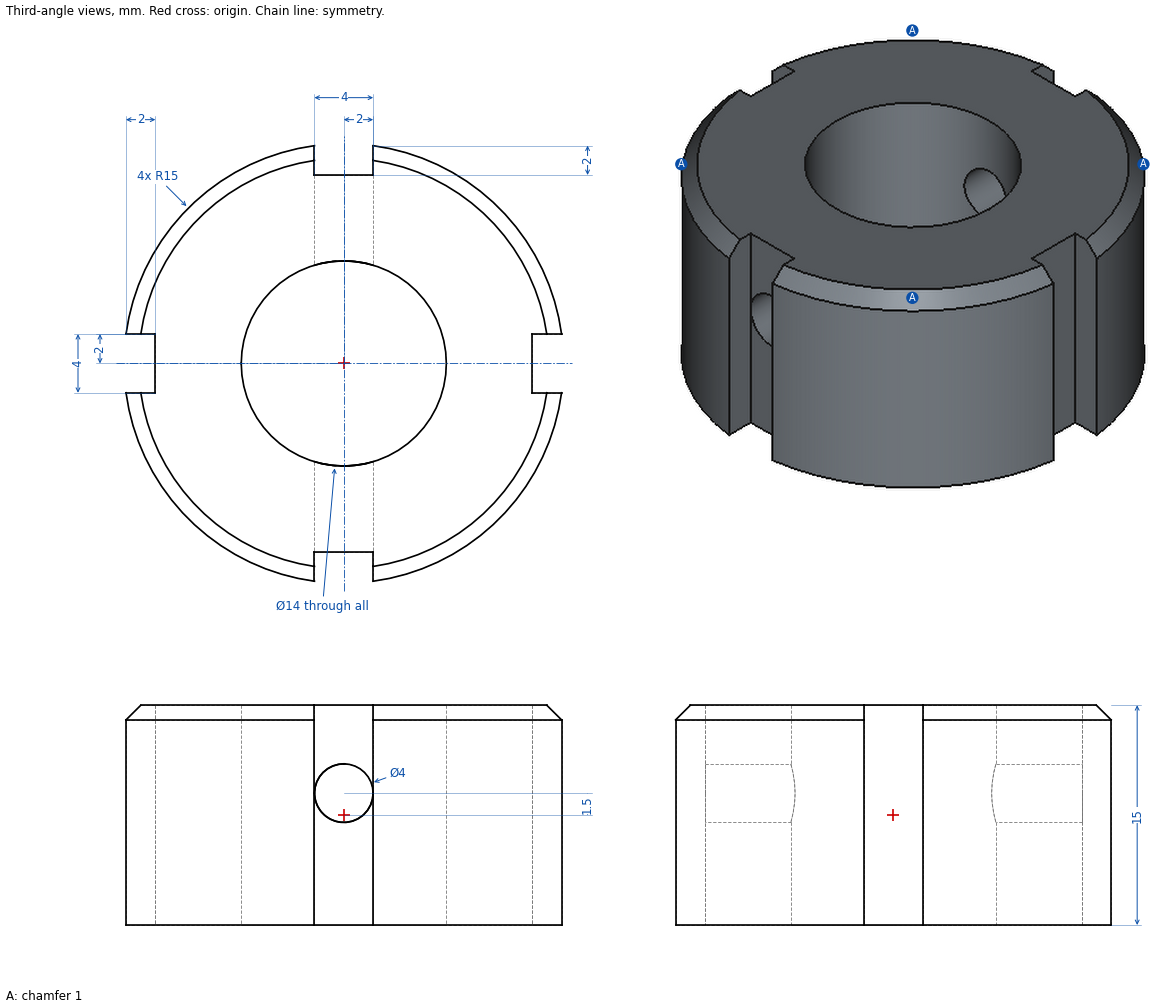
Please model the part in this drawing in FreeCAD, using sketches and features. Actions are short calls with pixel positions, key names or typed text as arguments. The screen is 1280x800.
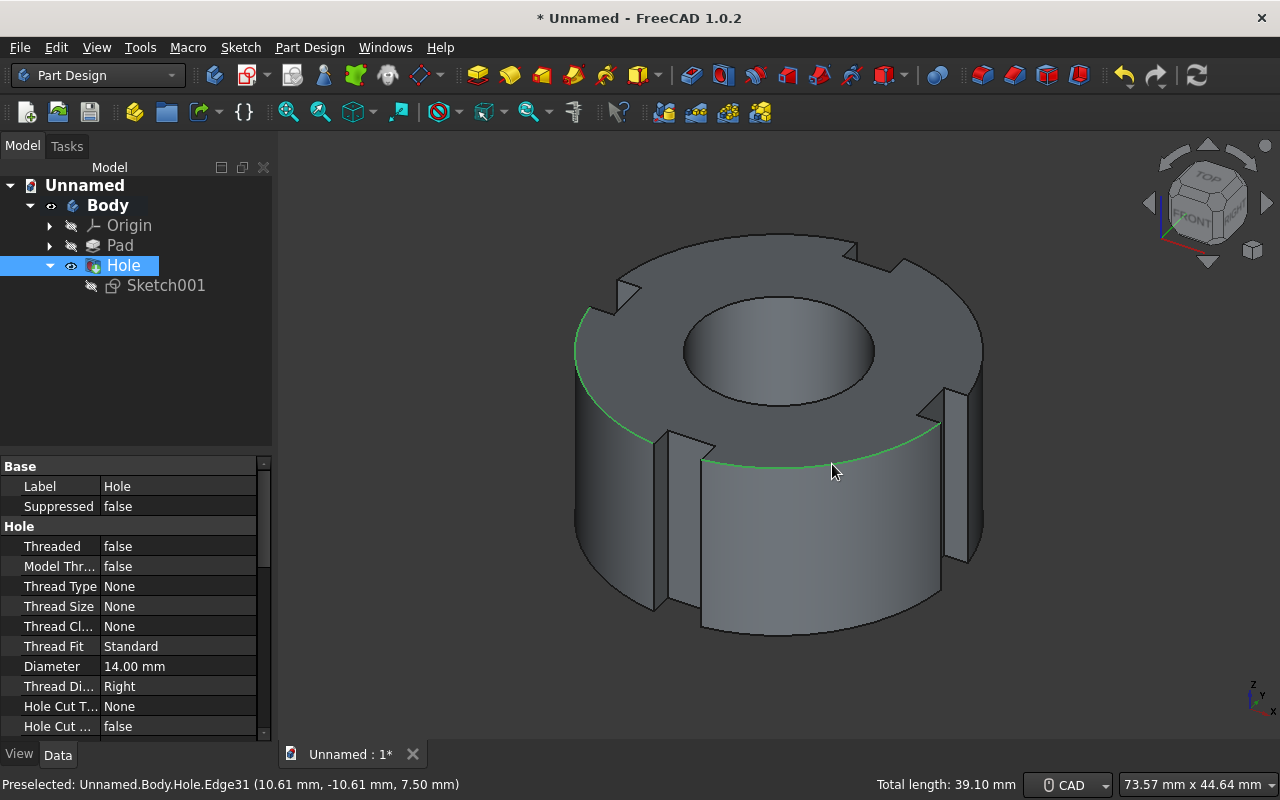
click(983, 350, ctrl)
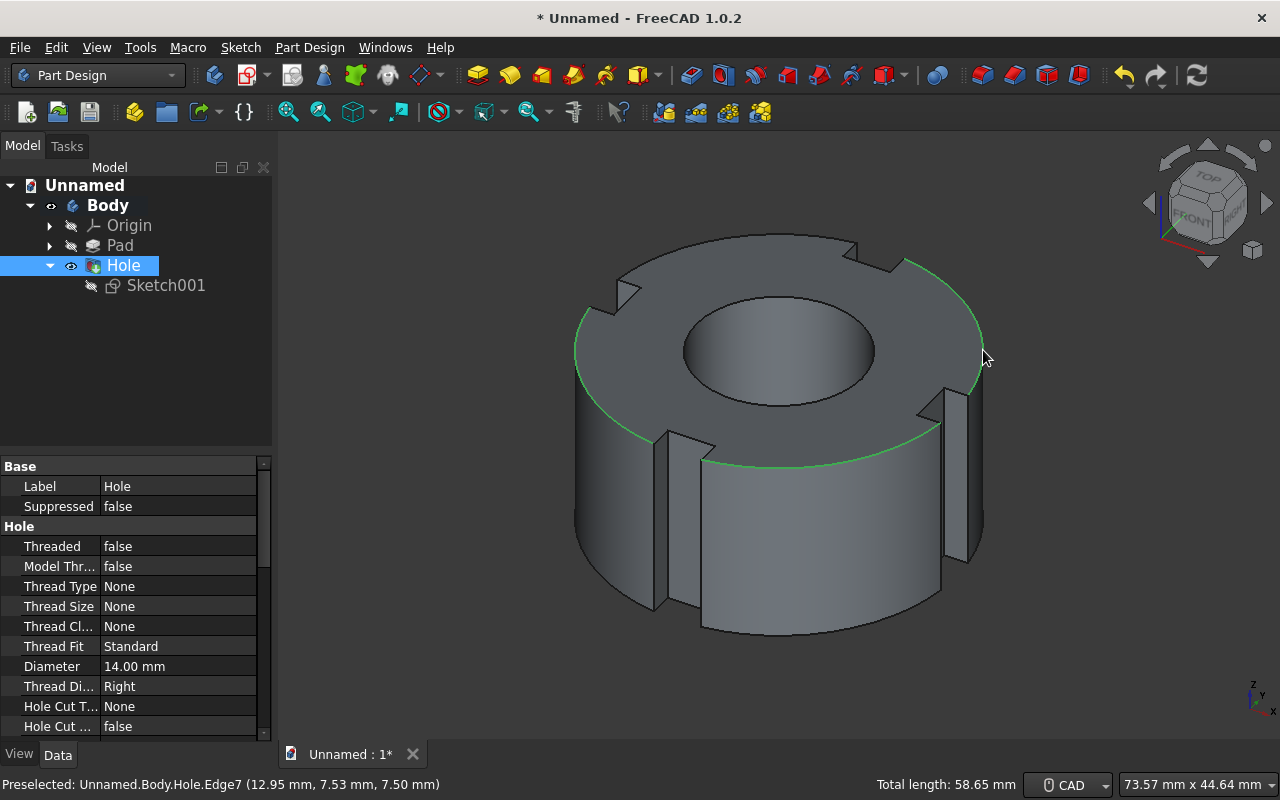
key(0)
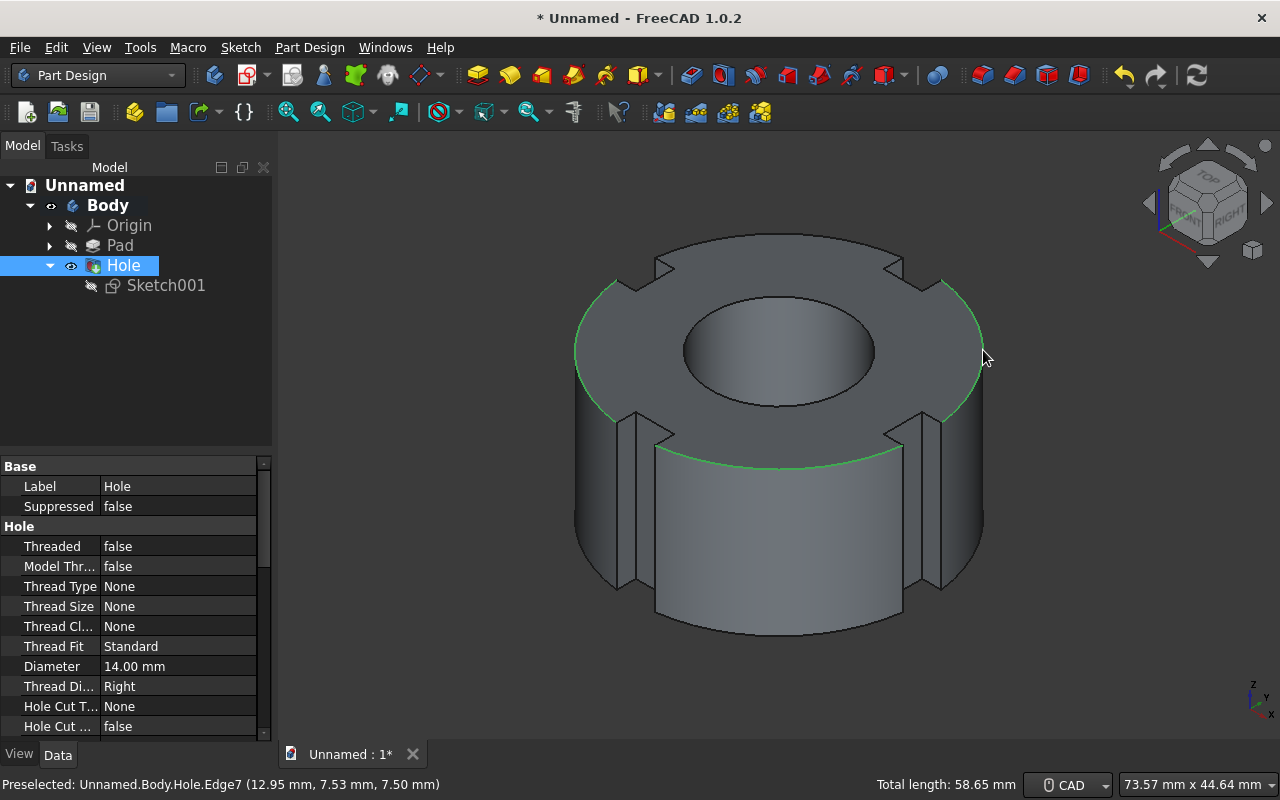
key(2)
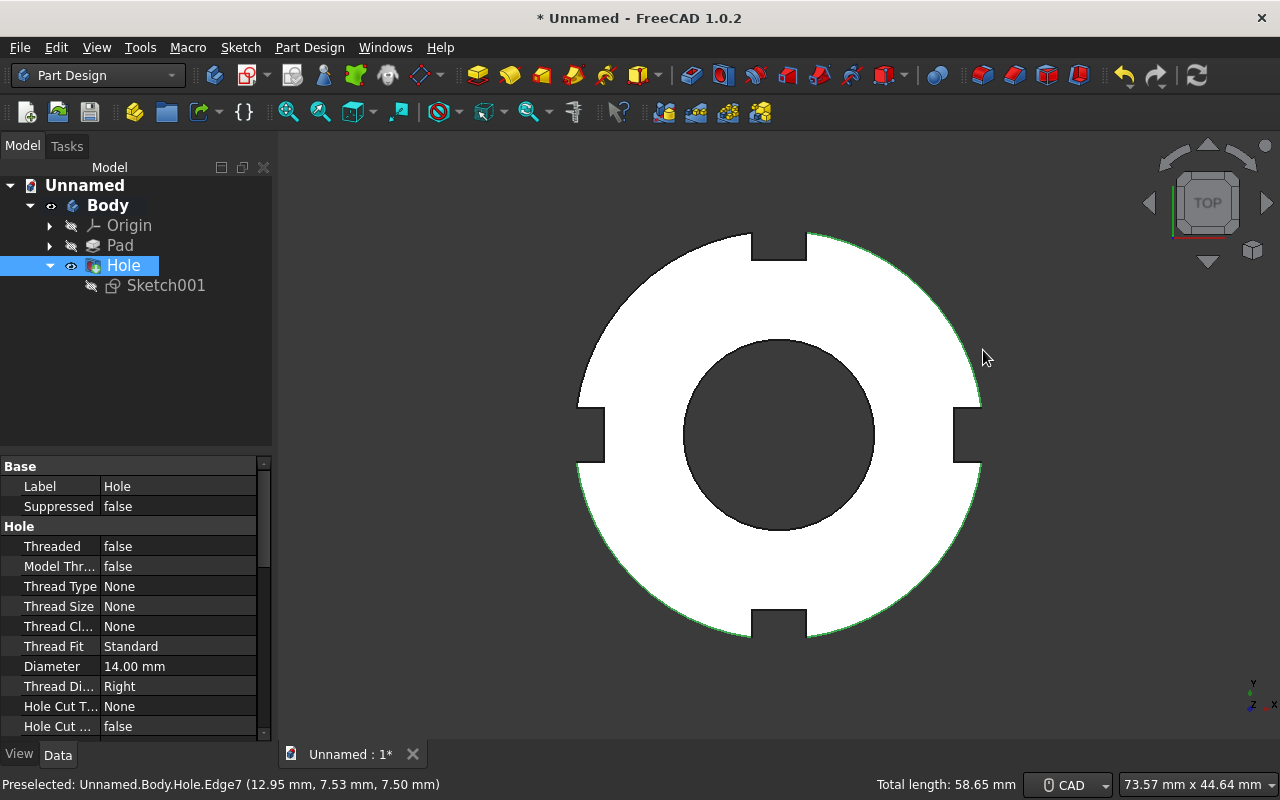
click(635, 290, ctrl)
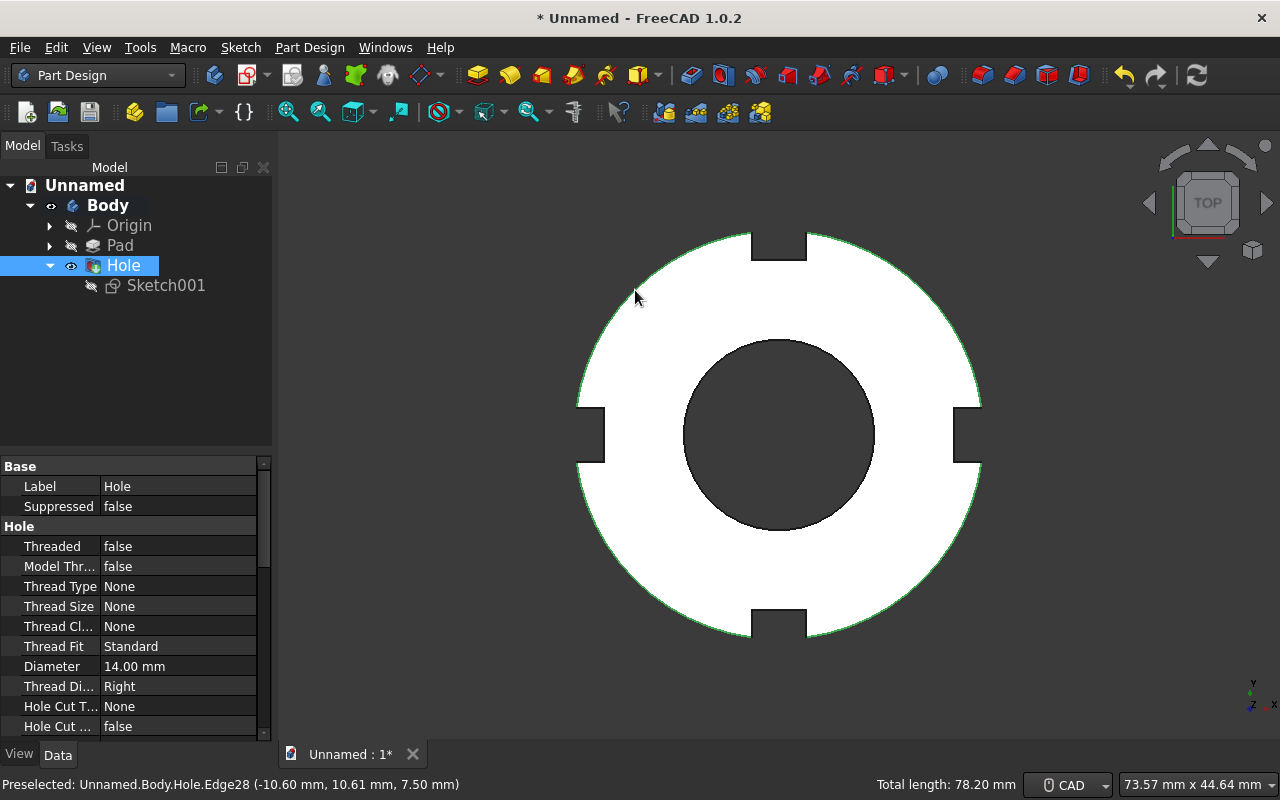
click(1016, 76)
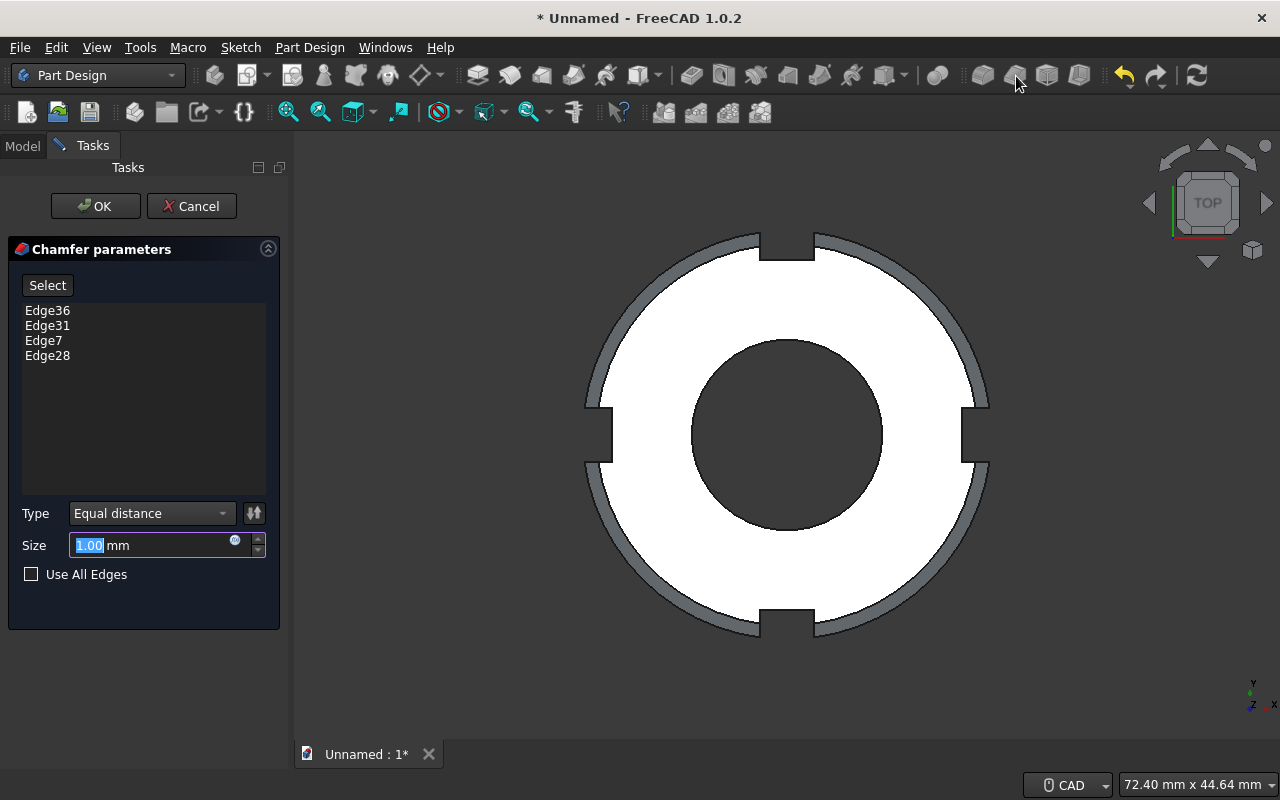
text(1)
key(Tab)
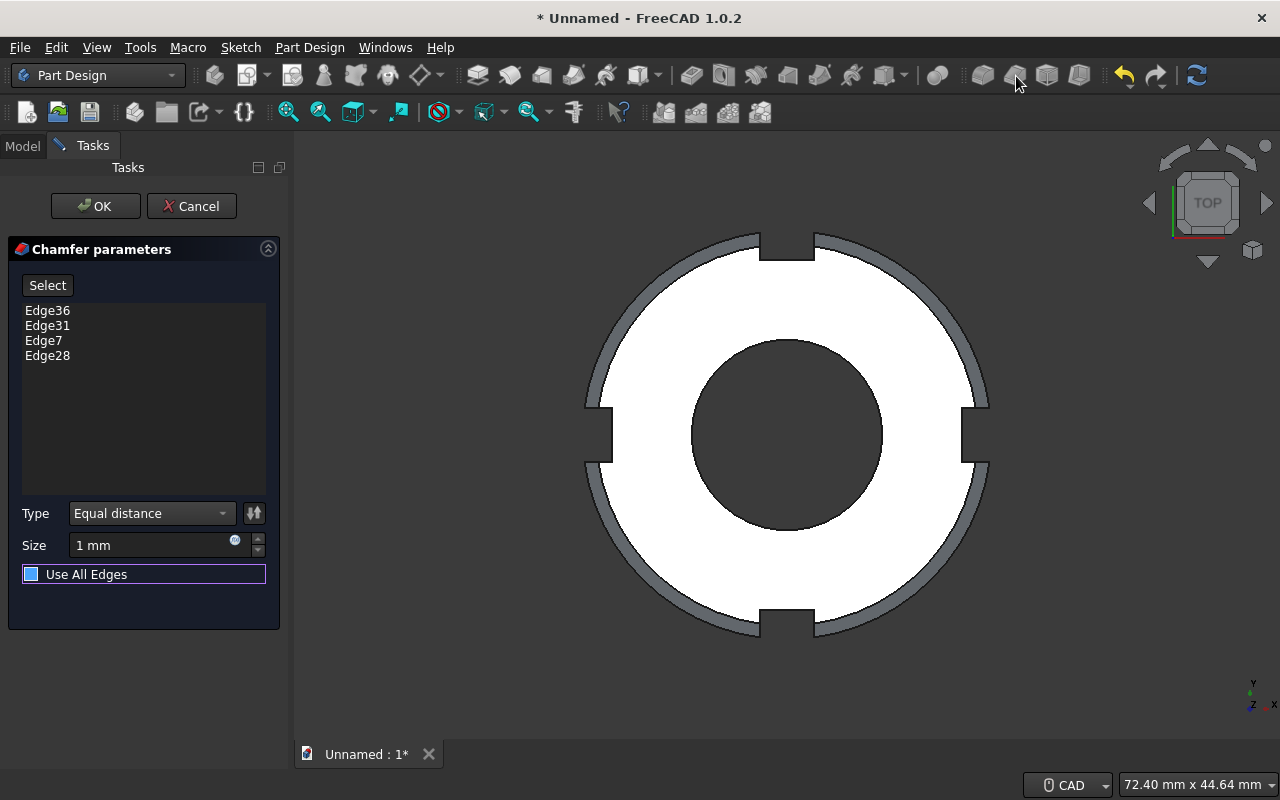
click(96, 206)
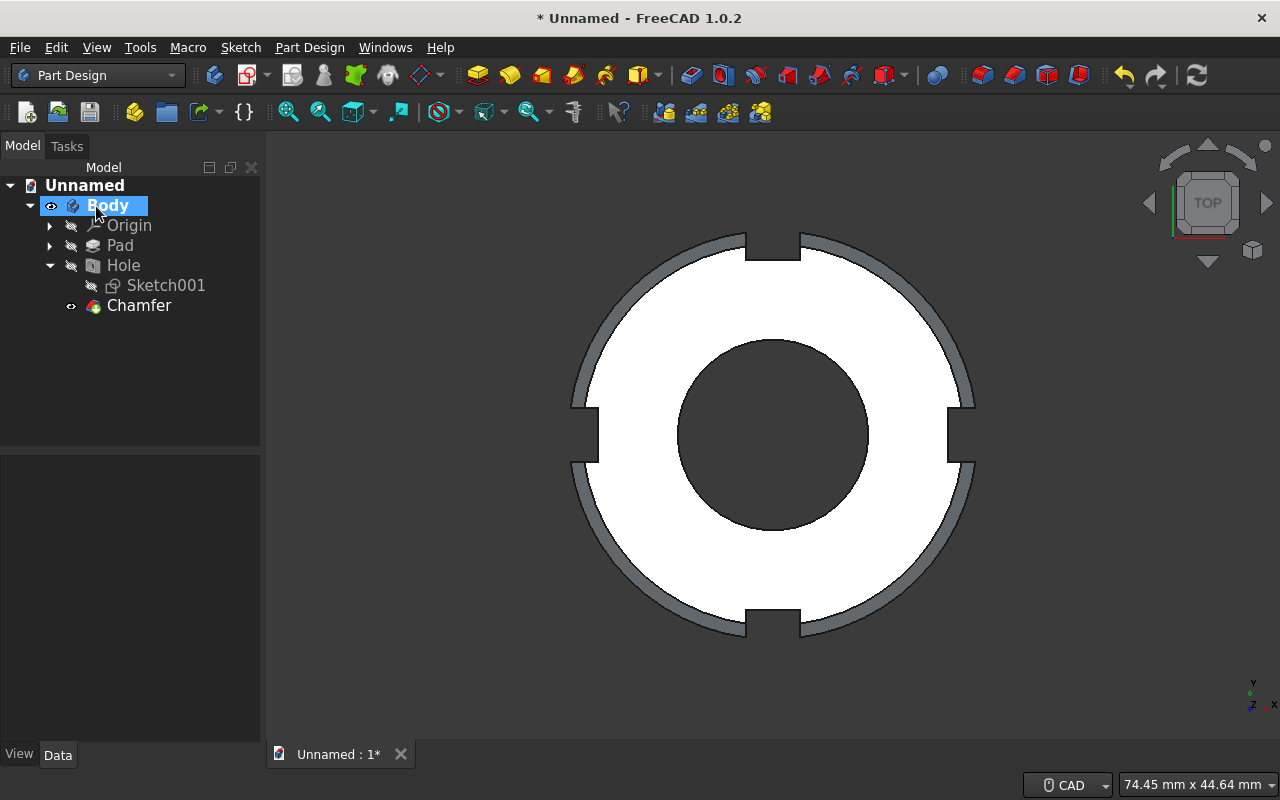
click(248, 76)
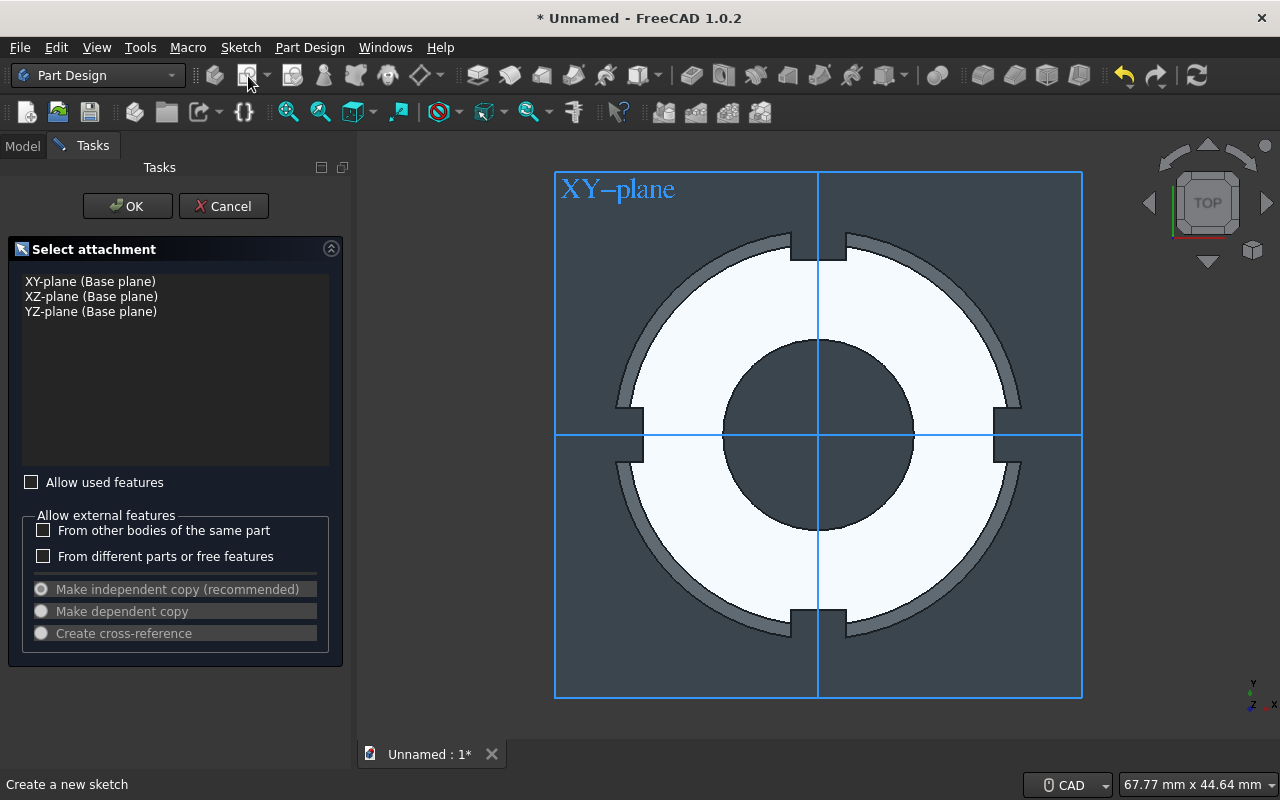
click(82, 296)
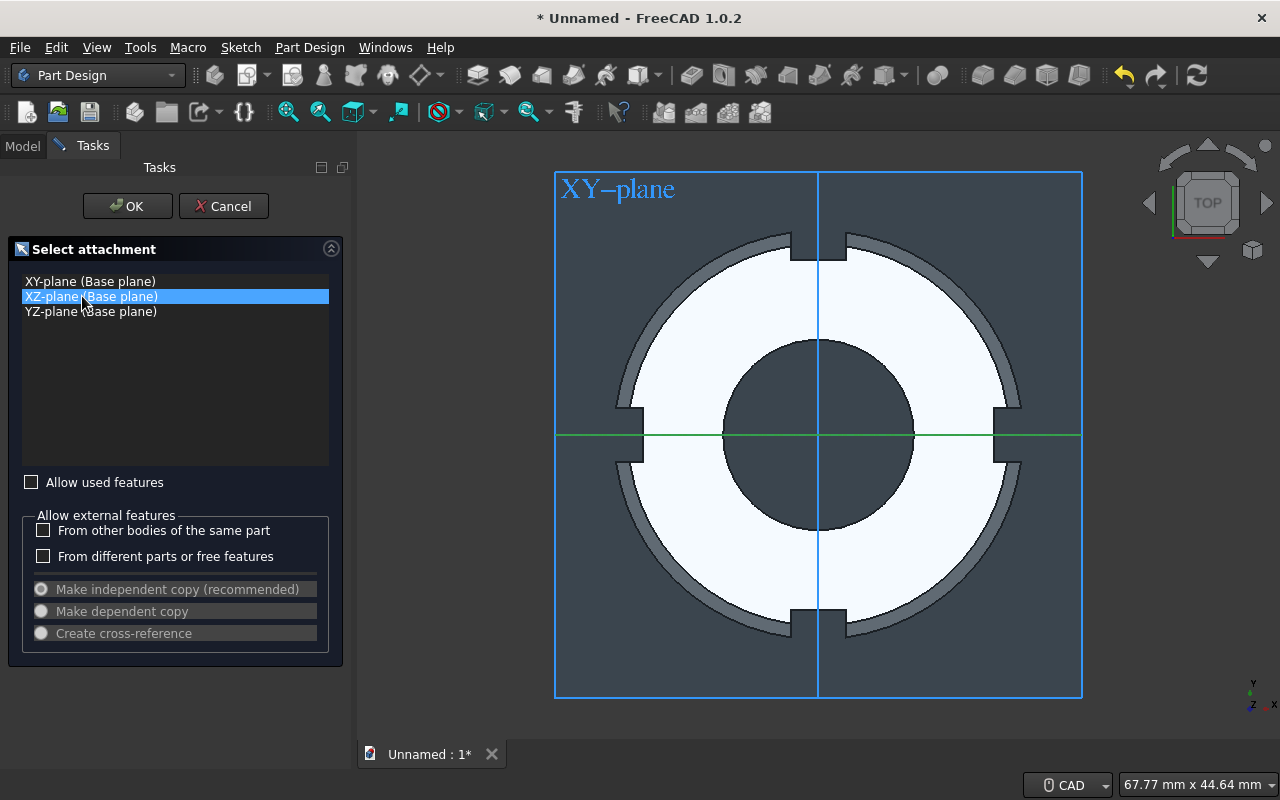
click(128, 206)